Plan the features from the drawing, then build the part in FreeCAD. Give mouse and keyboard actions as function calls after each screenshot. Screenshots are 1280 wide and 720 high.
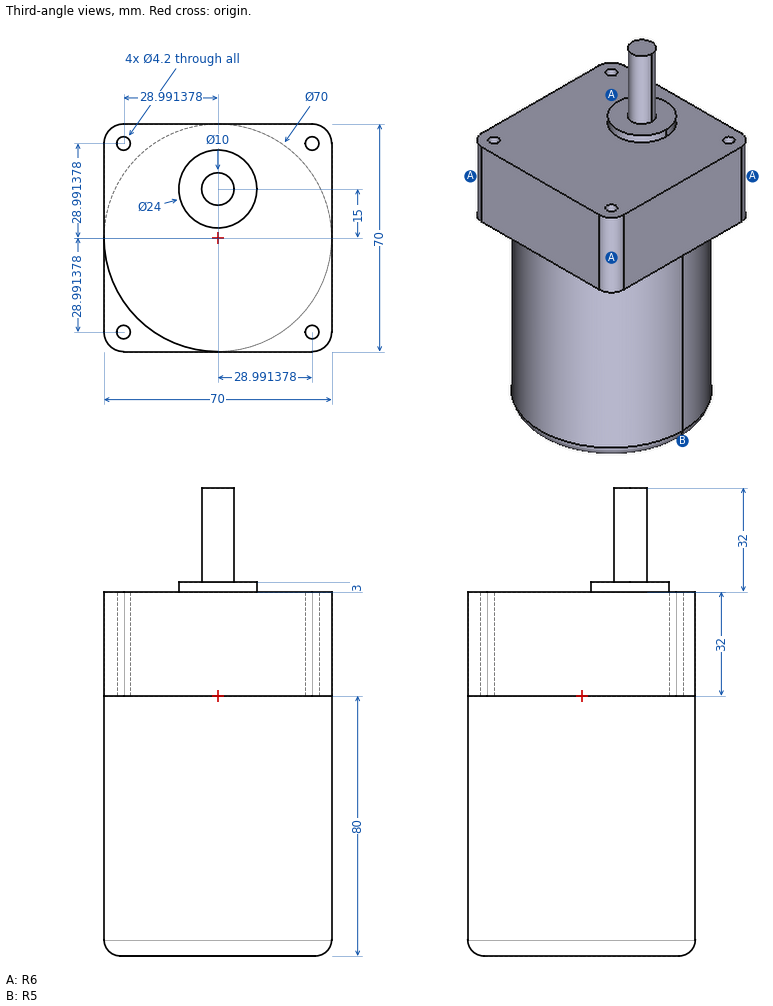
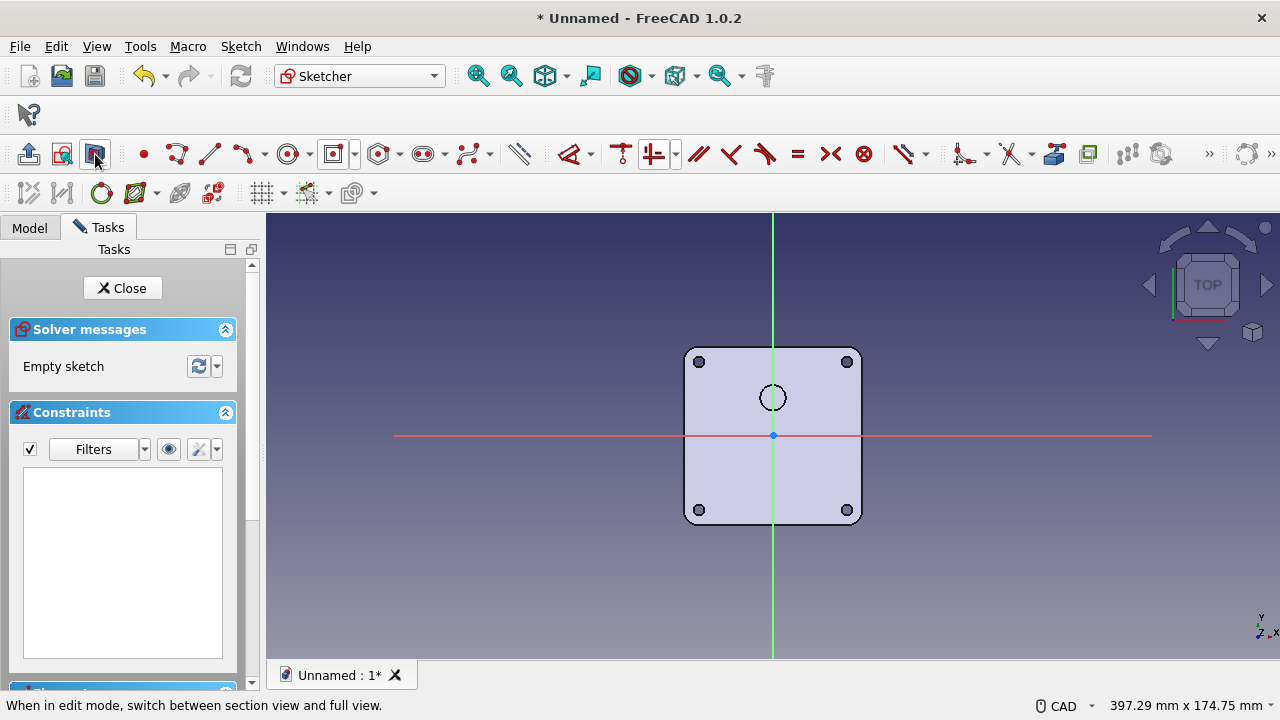
scroll(795, 390, up, 7)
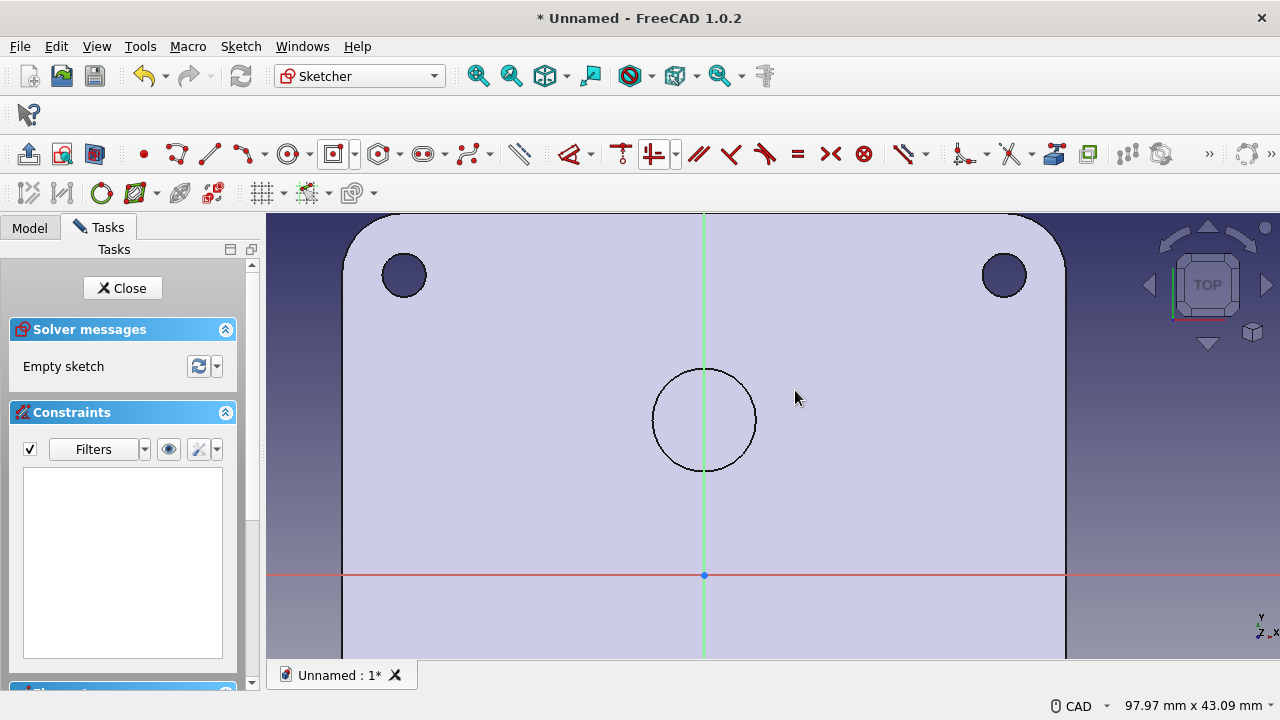
key(g)
key(c)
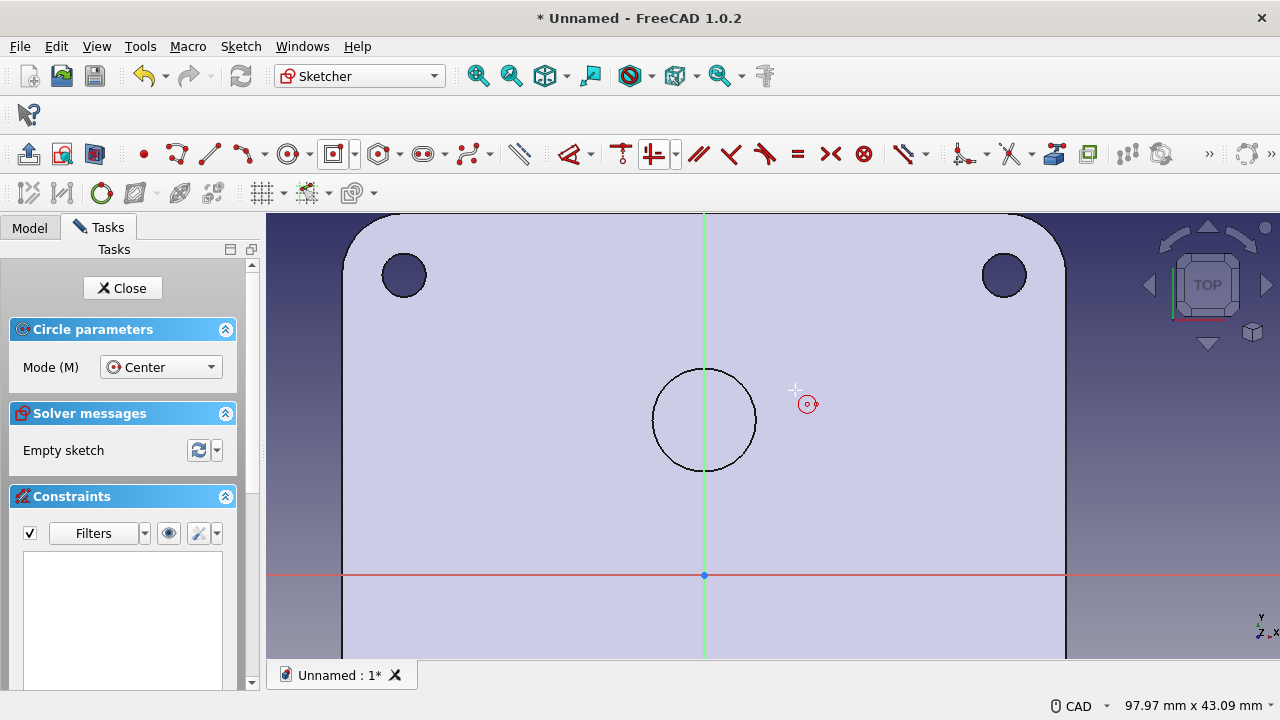
click(704, 420)
move(792, 332)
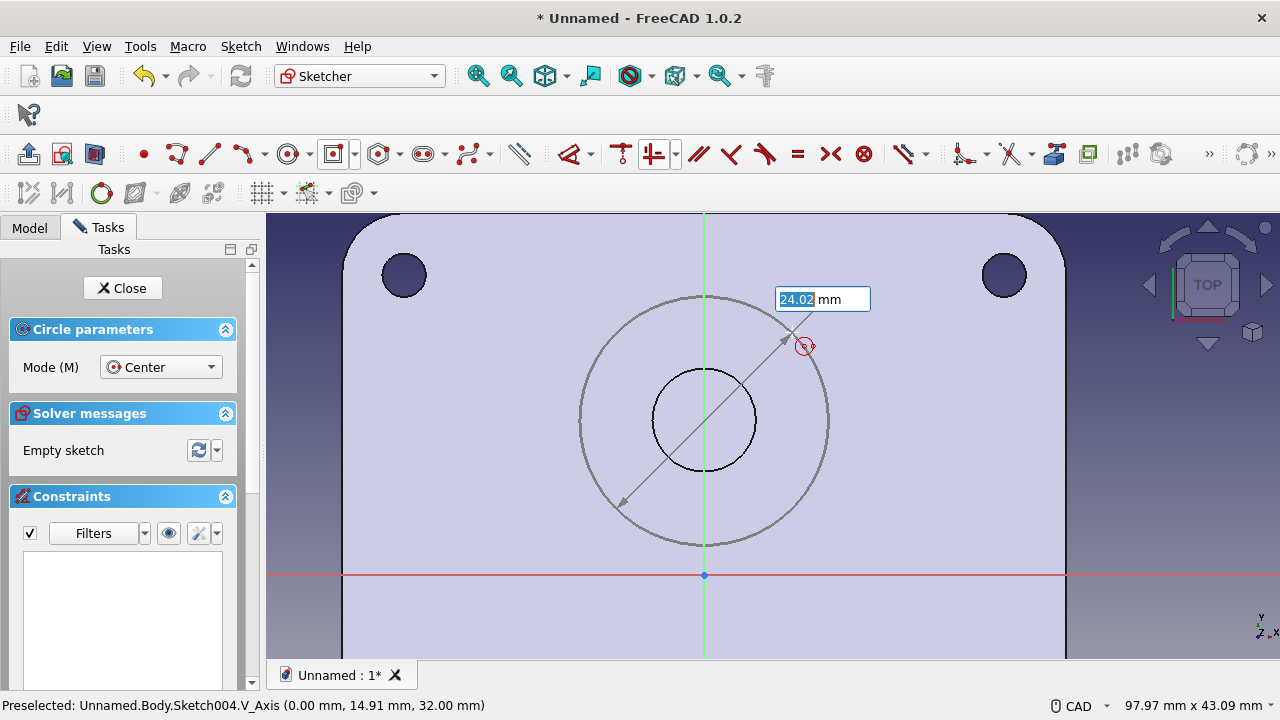
text(24)
key(Return)
key(Escape)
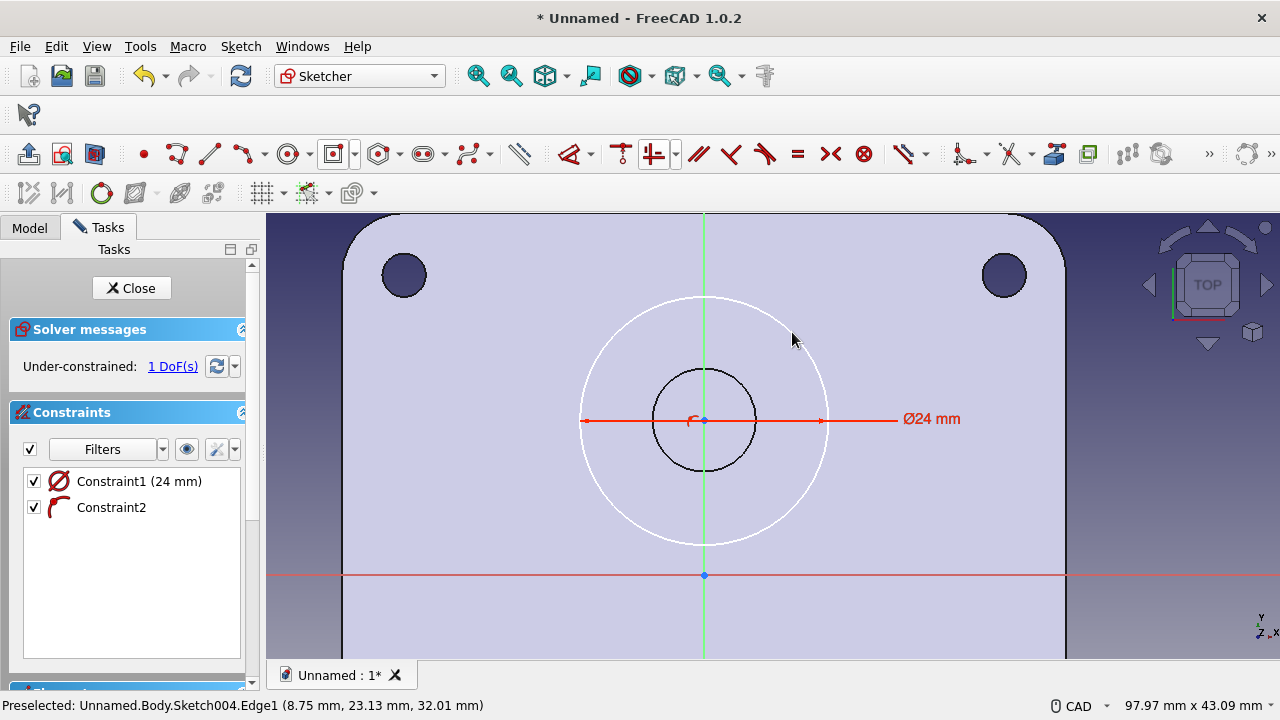
click(568, 154)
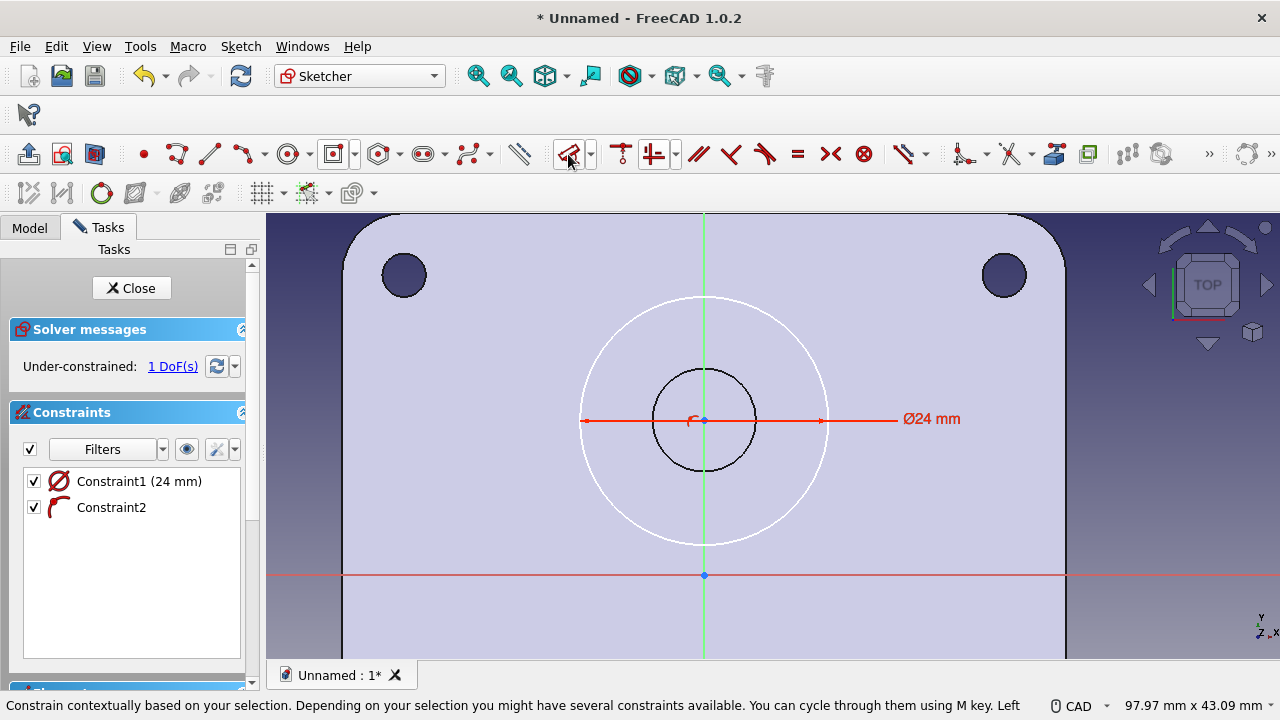
click(704, 421)
click(738, 498)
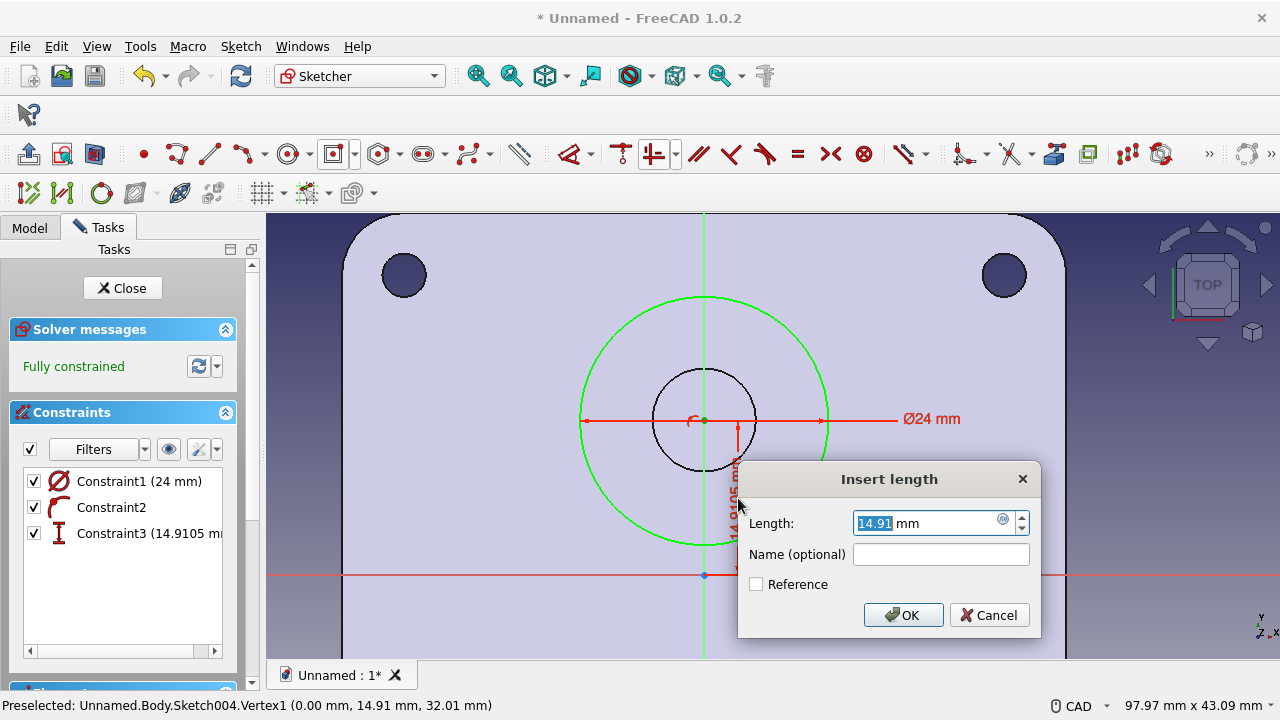
text(15)
key(Return)
key(Escape)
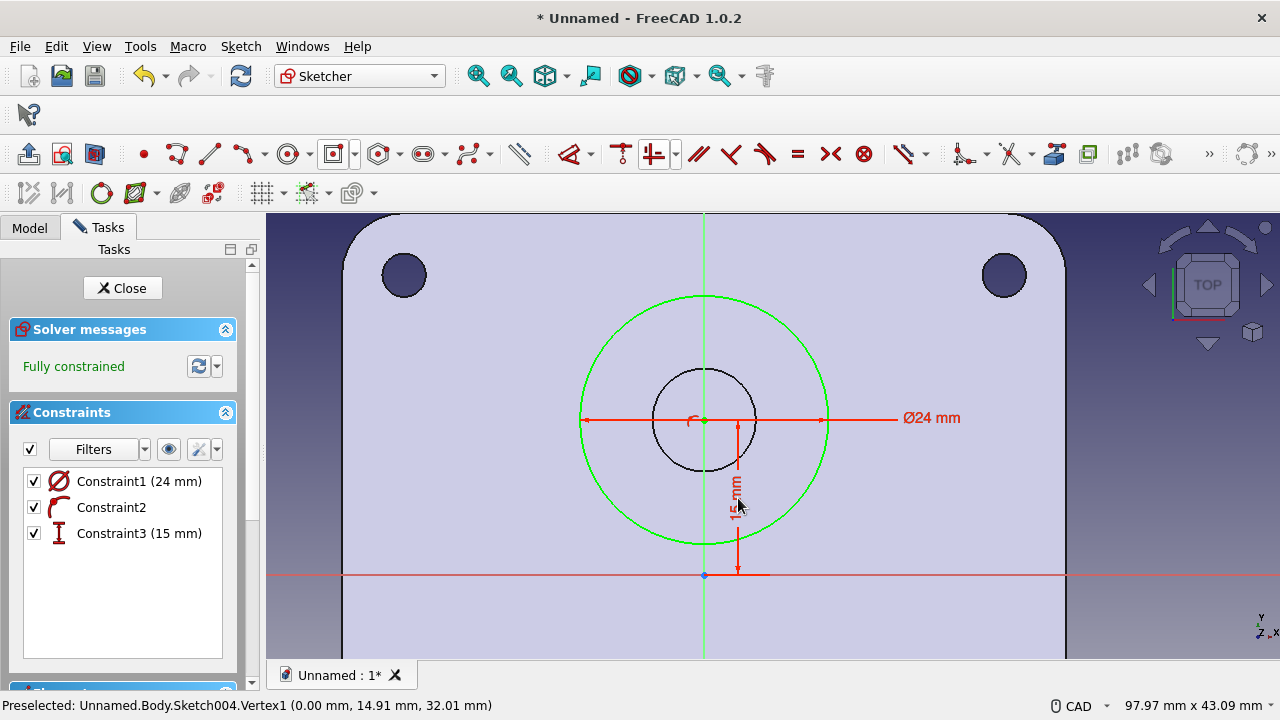
click(123, 288)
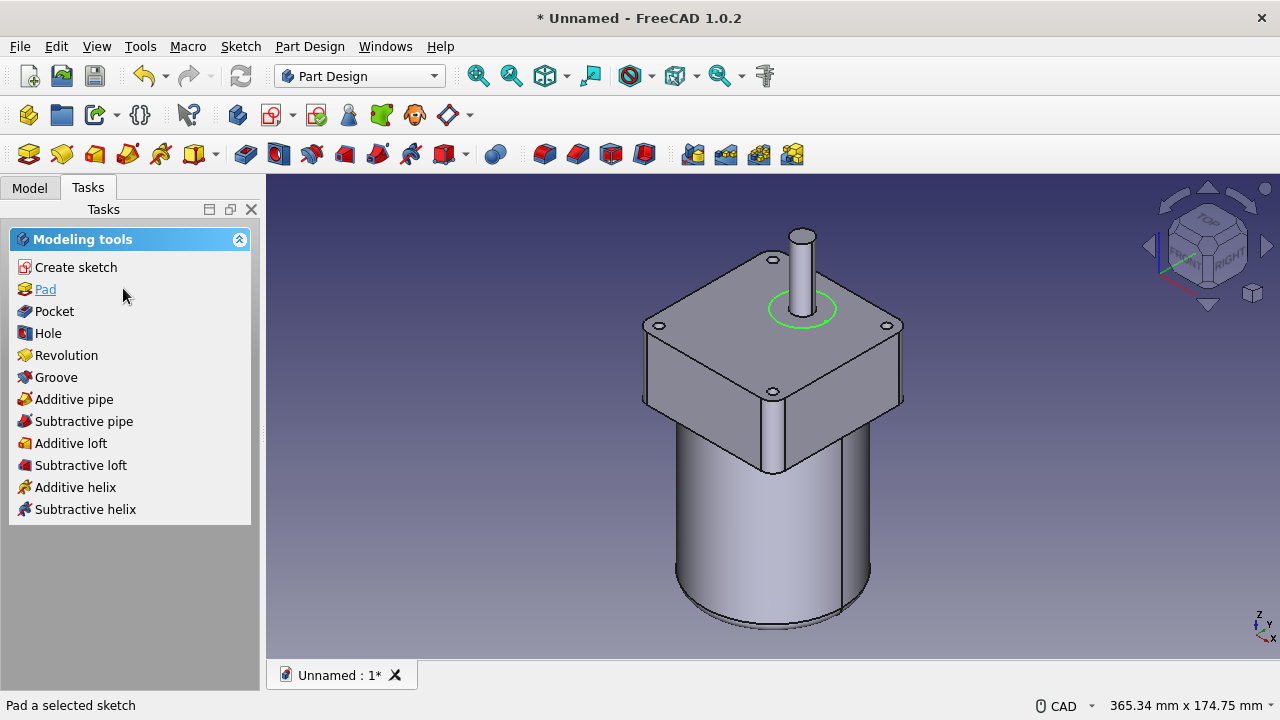
click(29, 154)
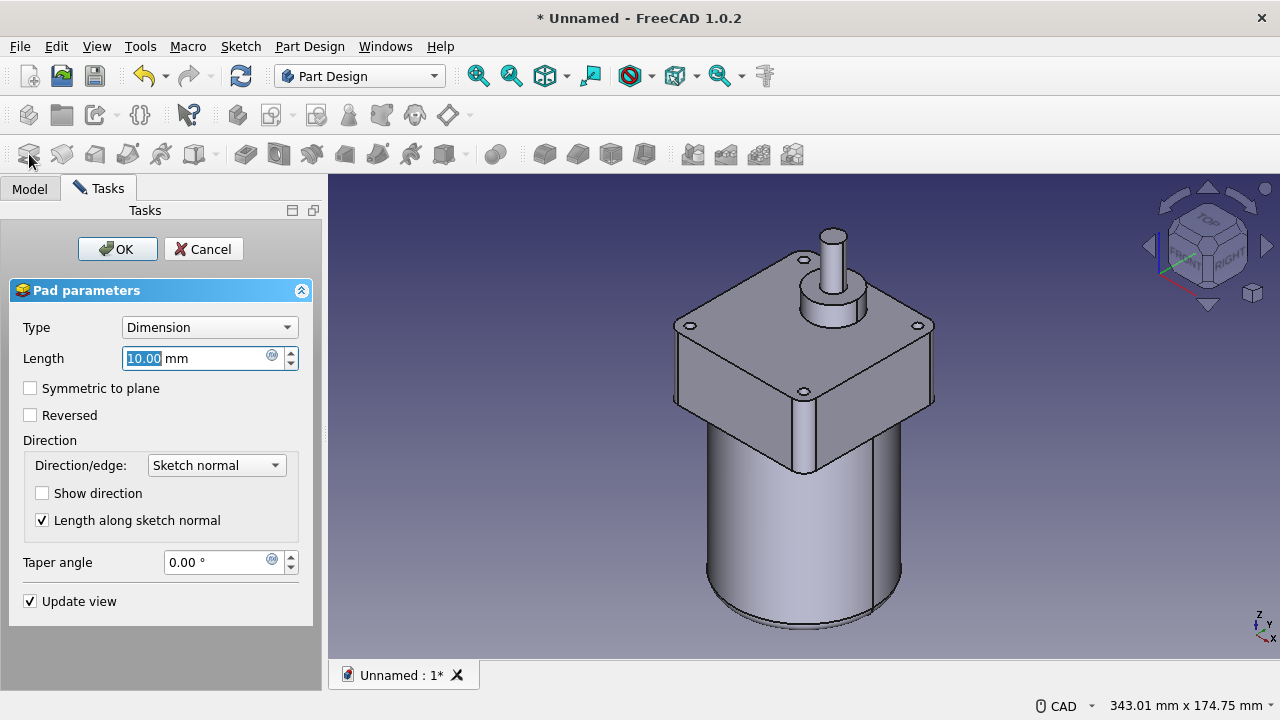
text(3)
key(Tab)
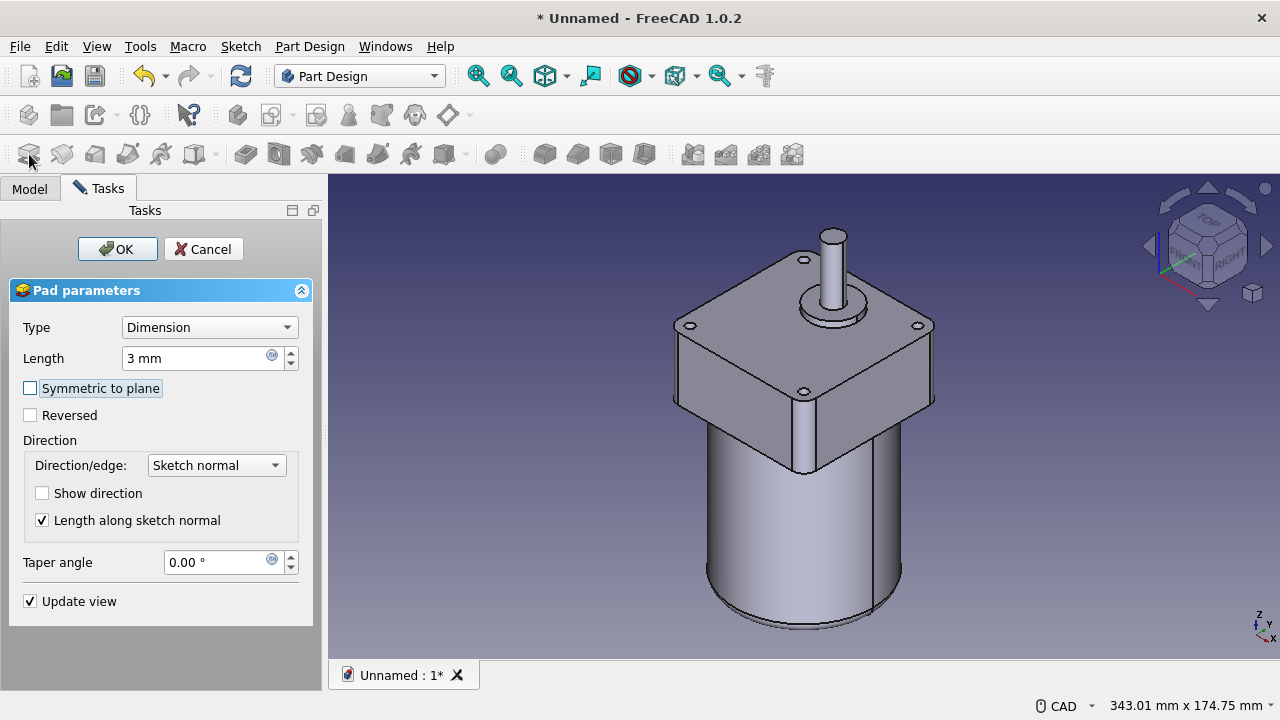
click(118, 249)